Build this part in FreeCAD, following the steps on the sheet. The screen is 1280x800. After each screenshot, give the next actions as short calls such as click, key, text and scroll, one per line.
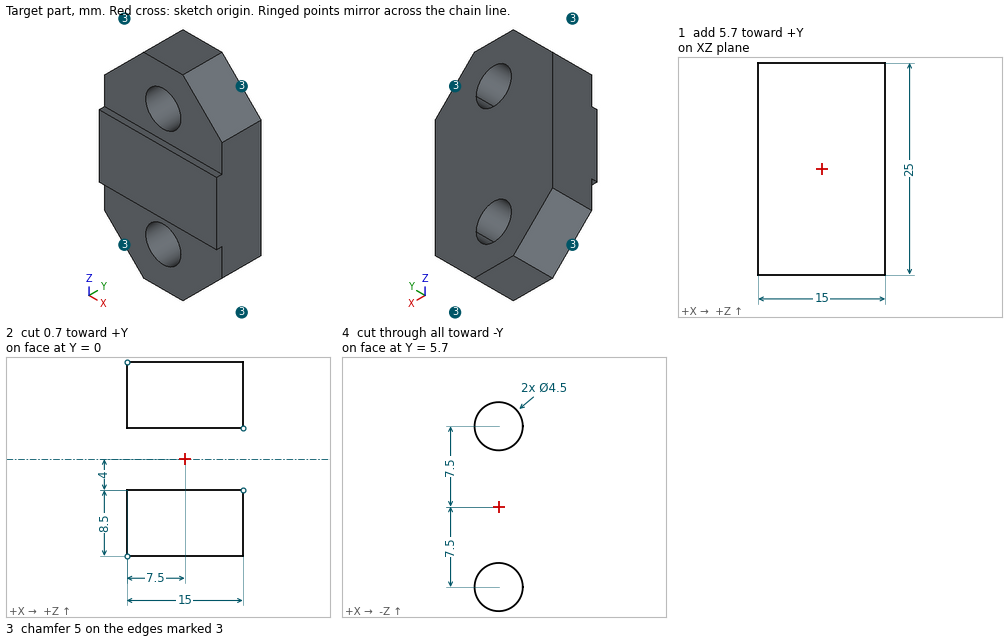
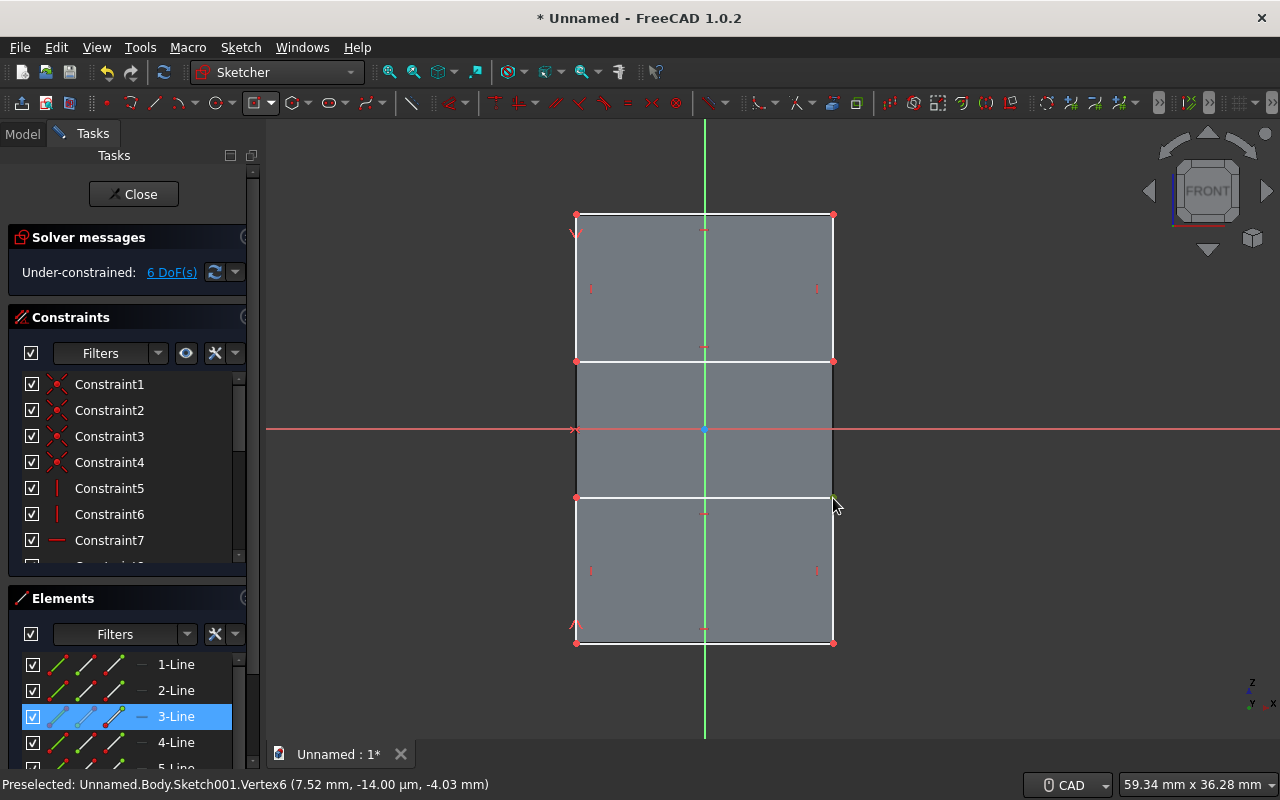
click(833, 362)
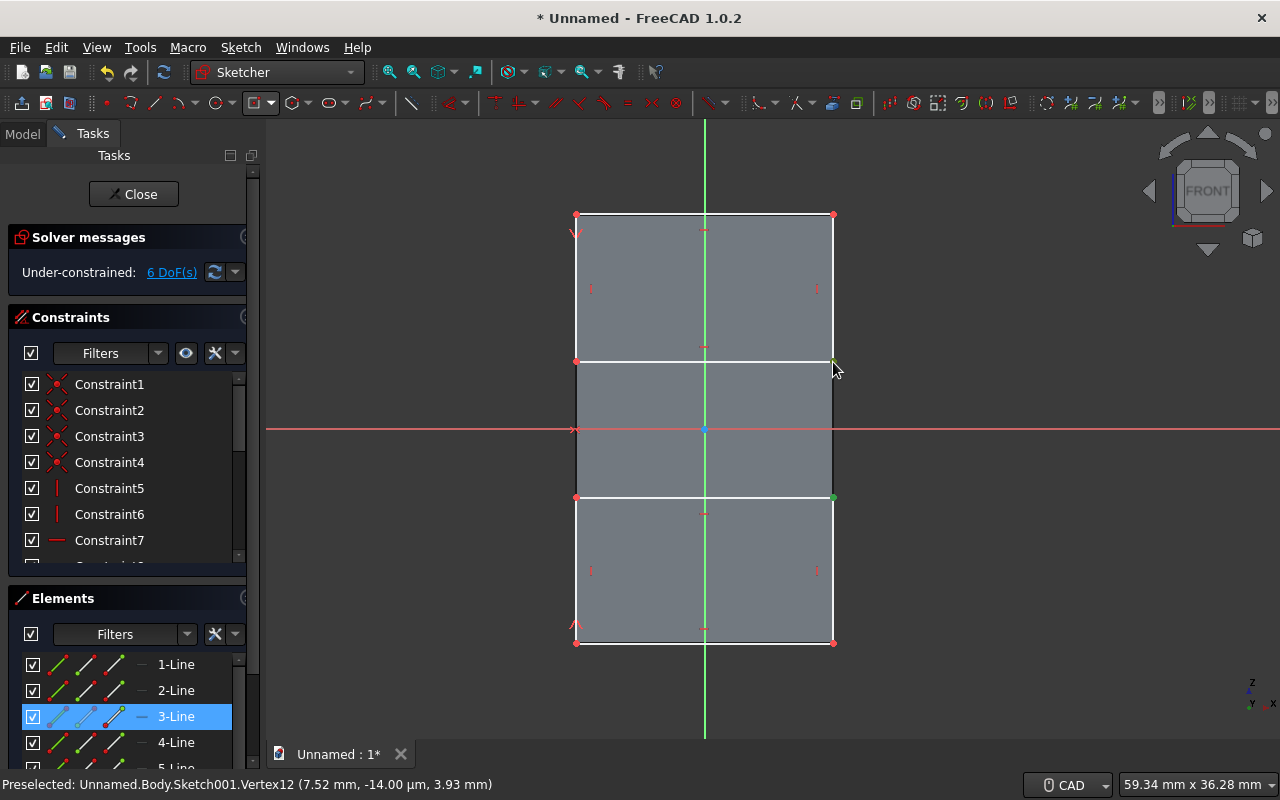
click(353, 429)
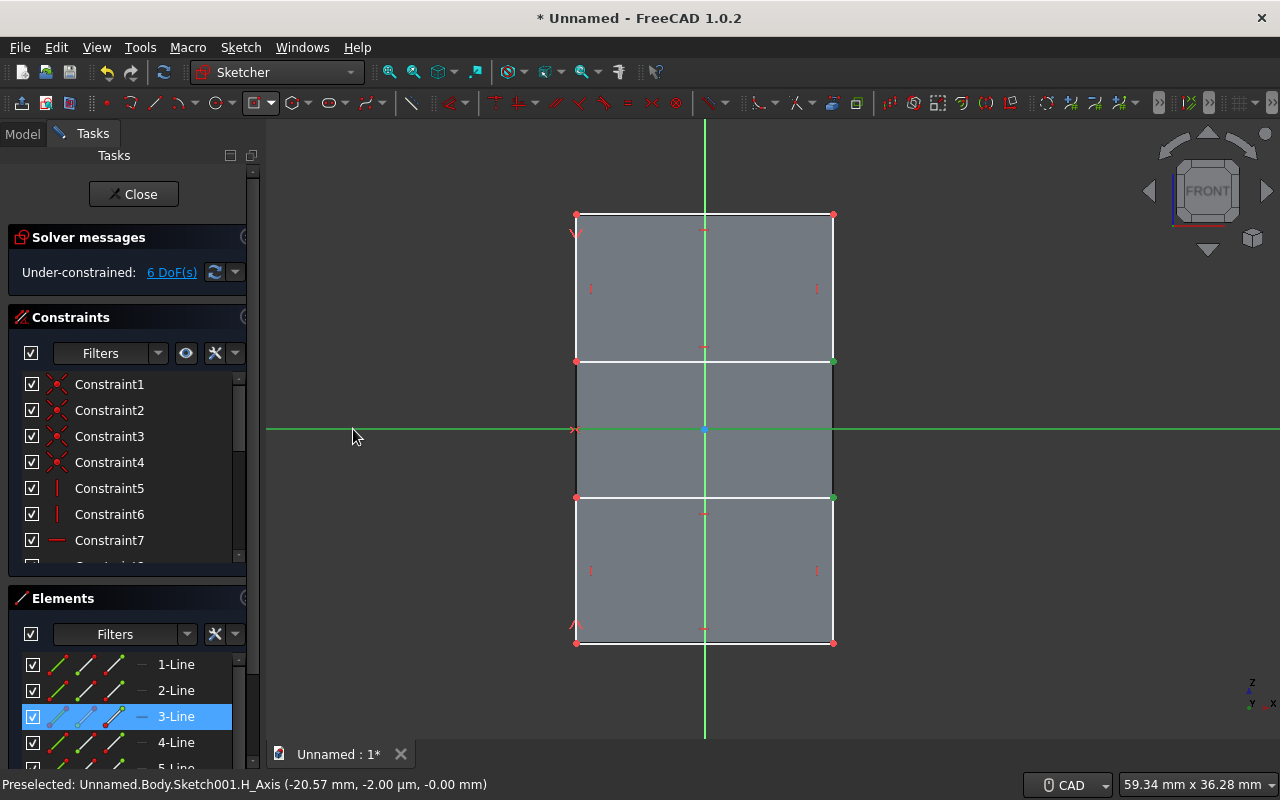
key(s)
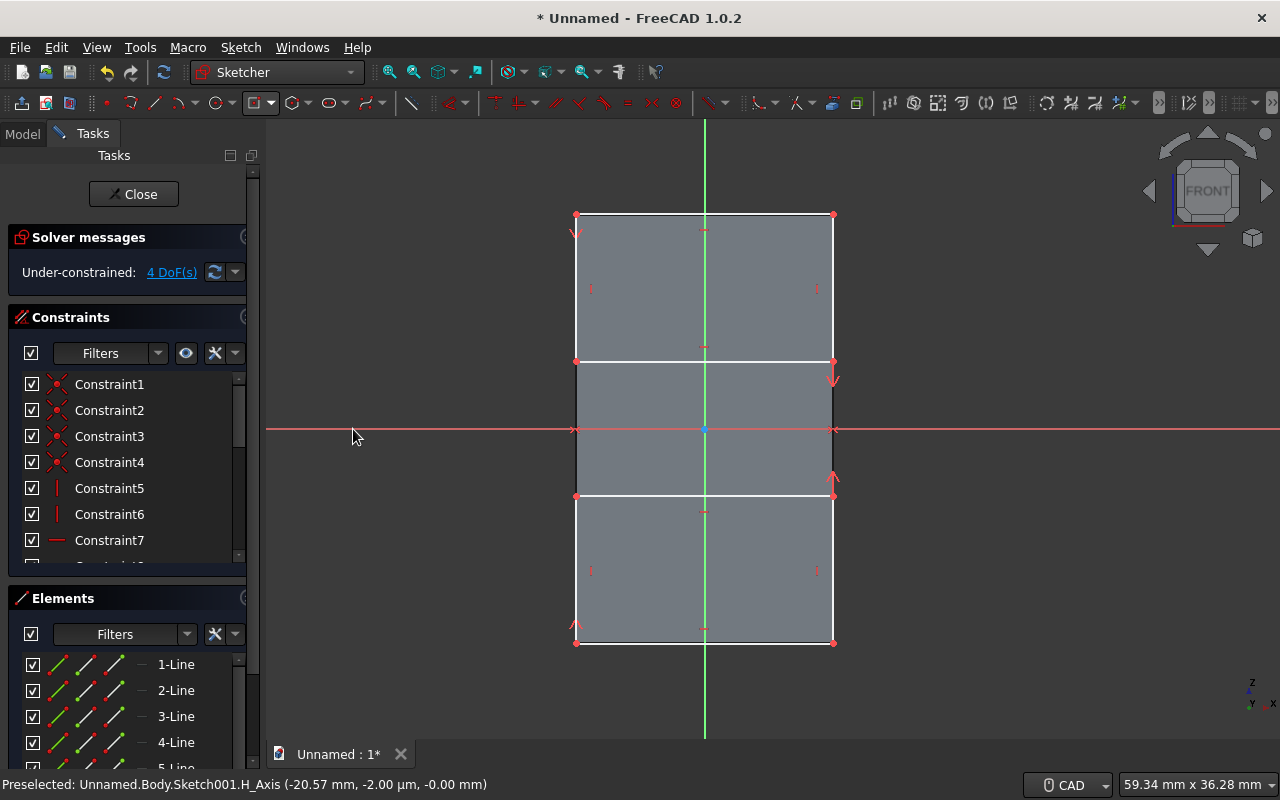
key(d)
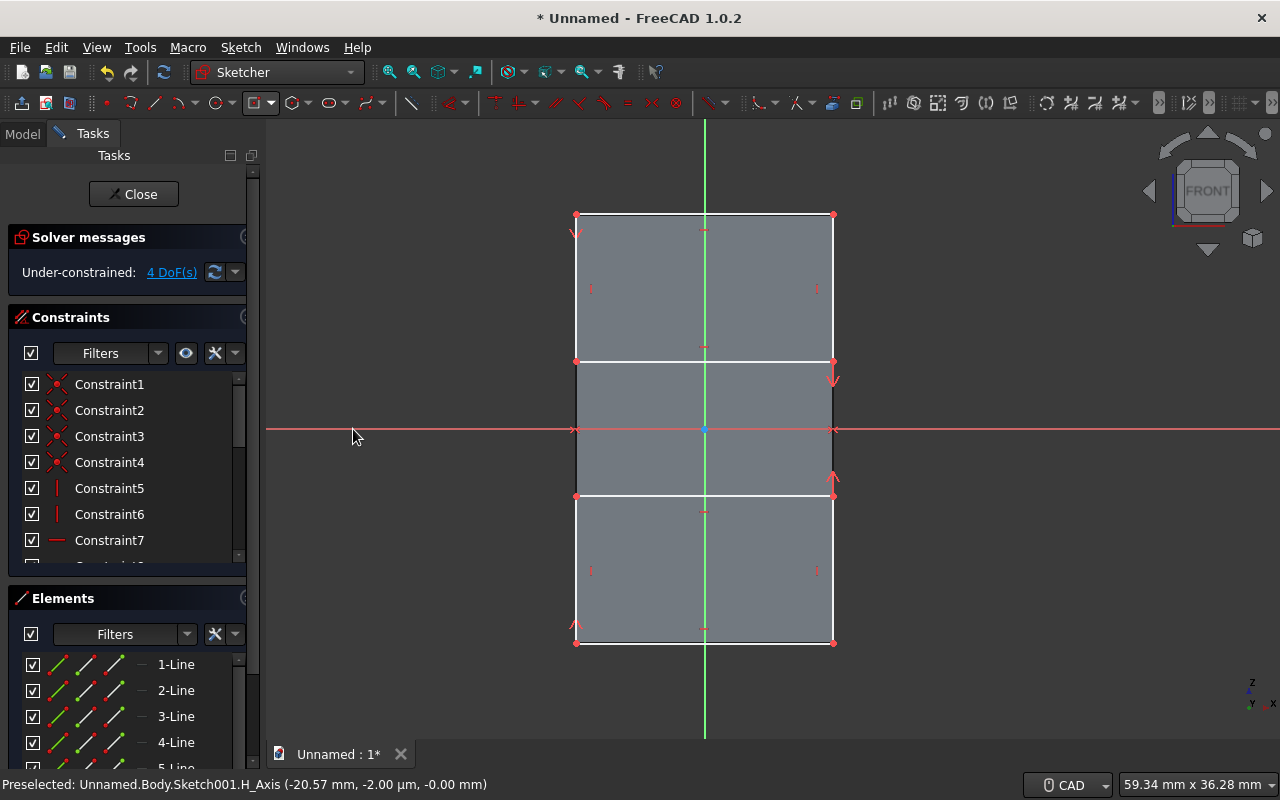
click(653, 644)
click(645, 678)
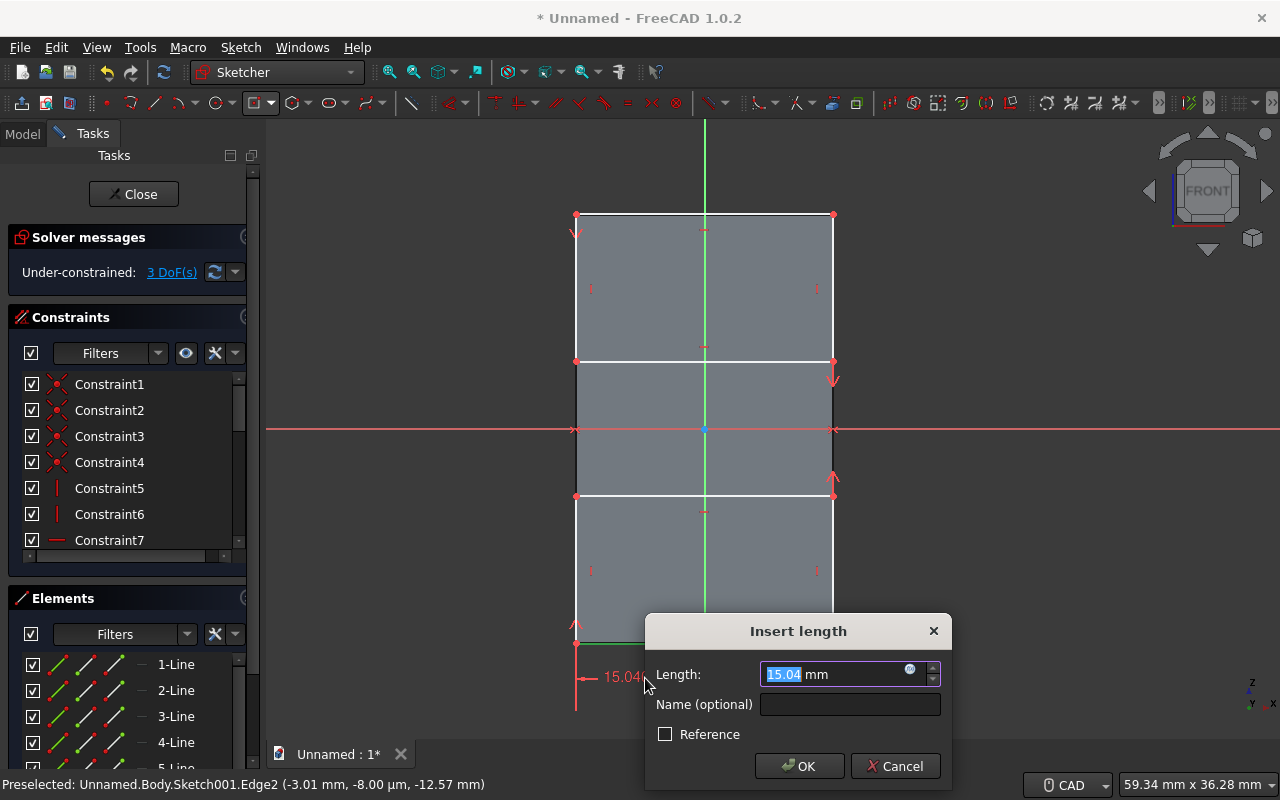
text(15)
key(Return)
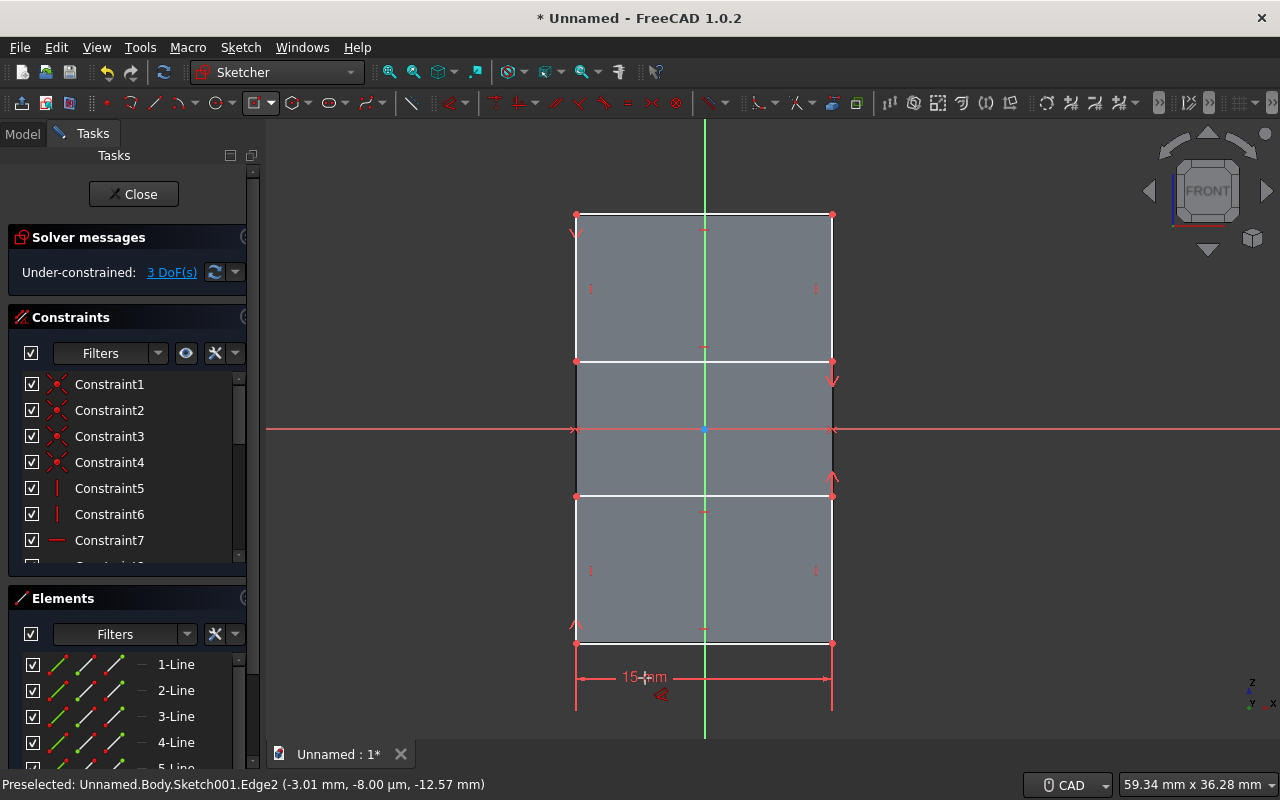
click(576, 496)
click(542, 463)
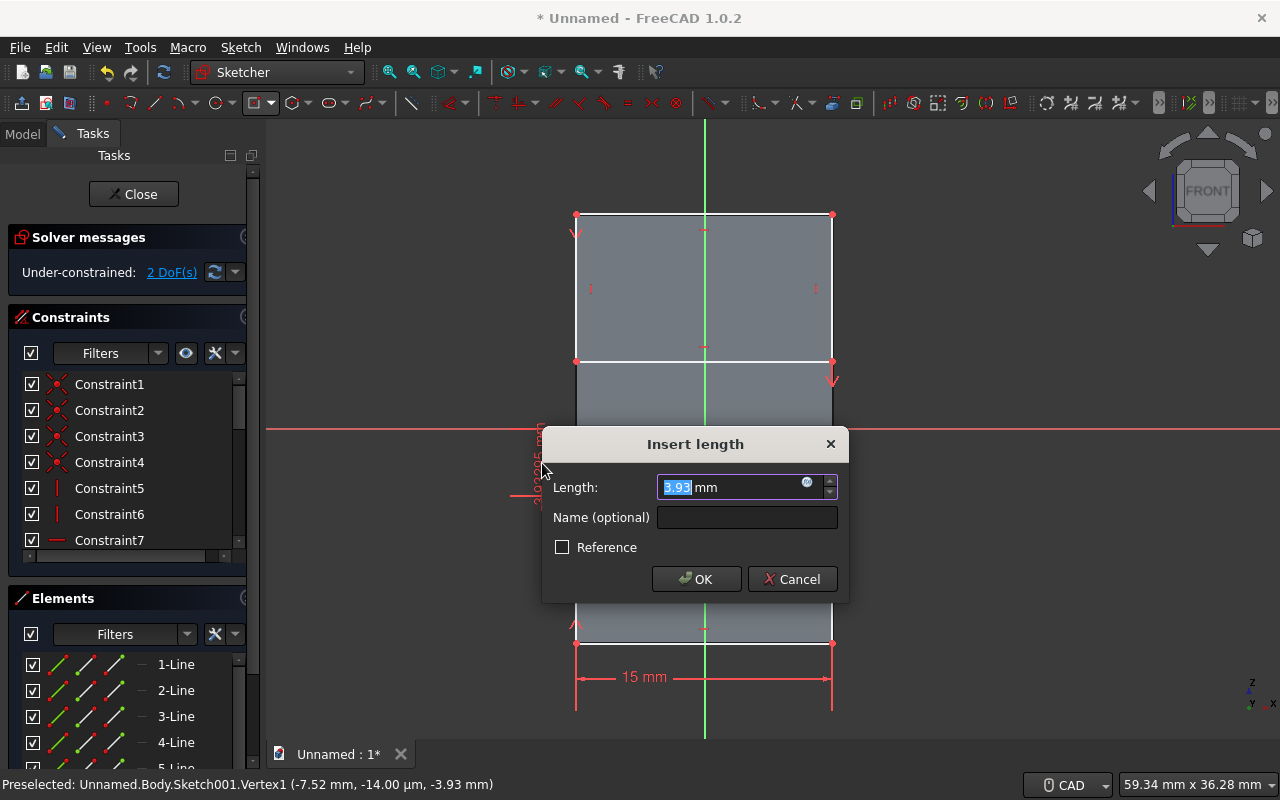
text(4)
key(Return)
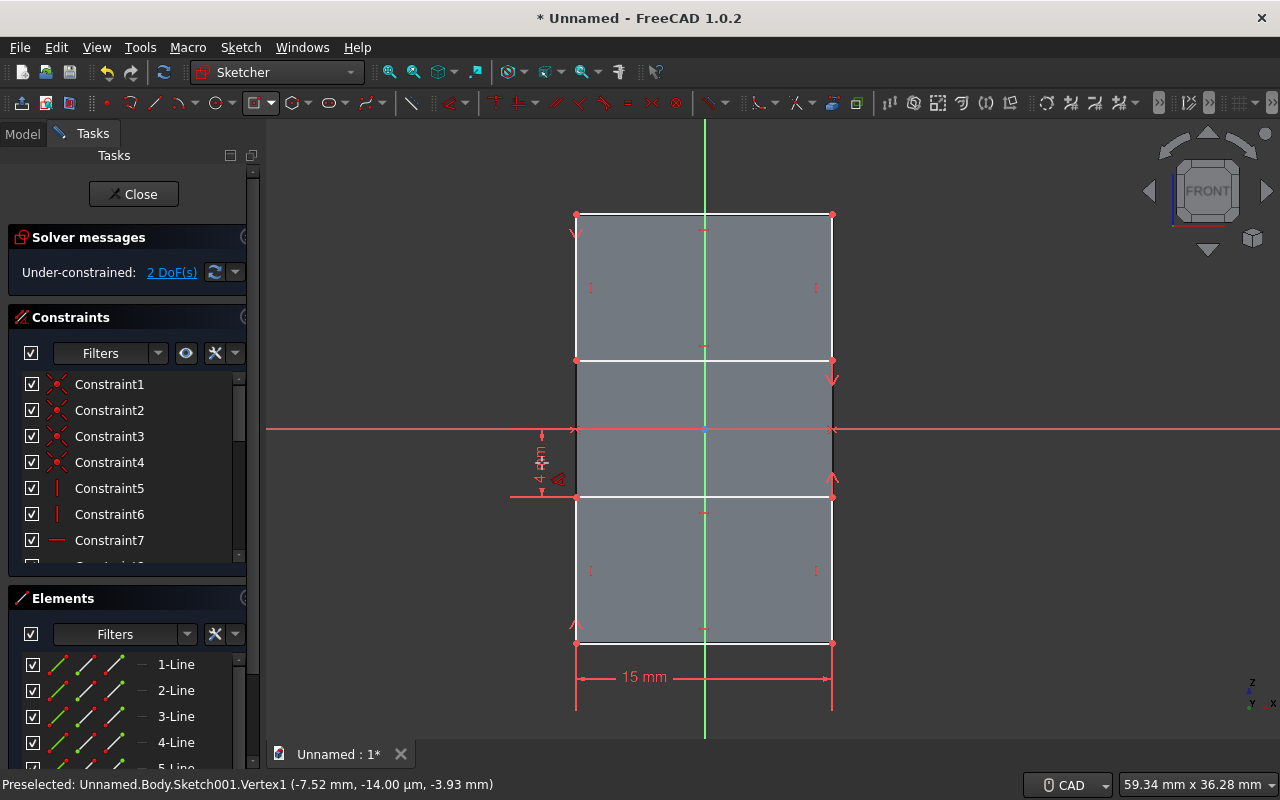
click(576, 541)
click(542, 571)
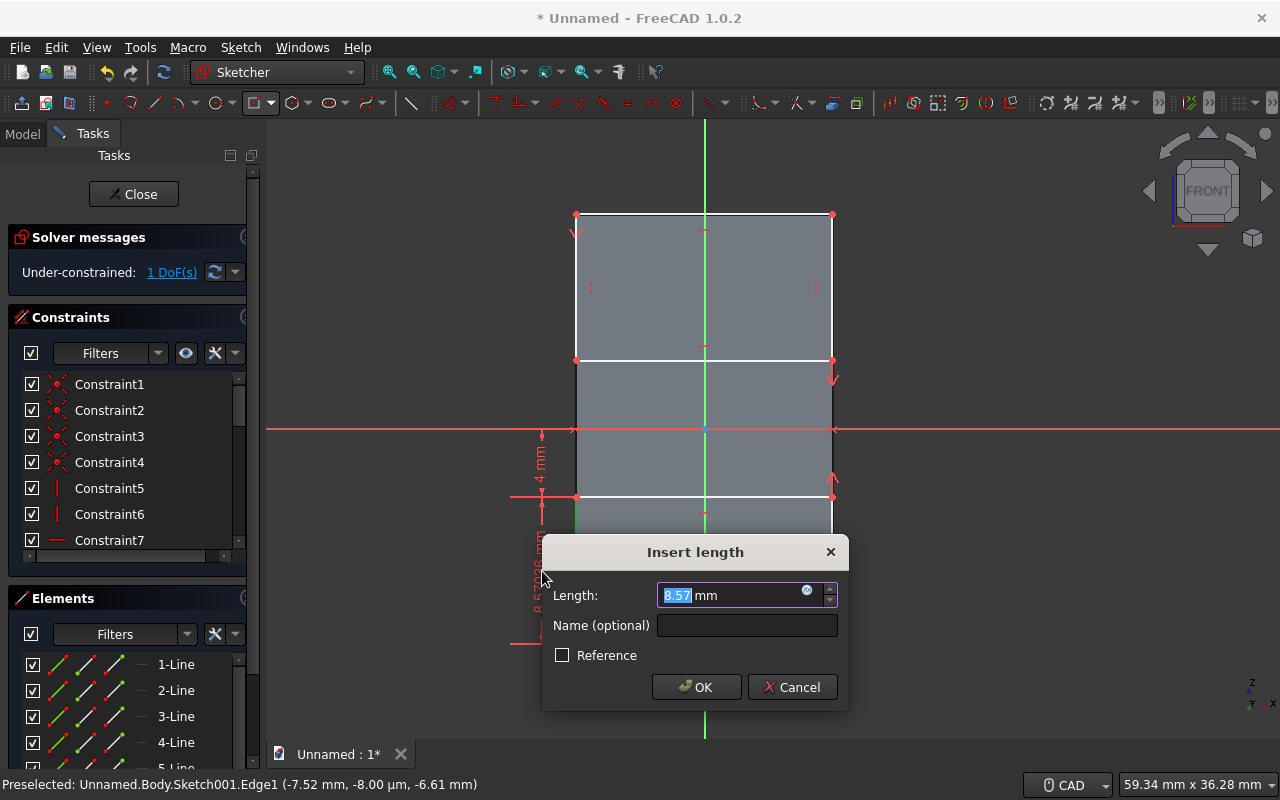
text(8.5)
key(Return)